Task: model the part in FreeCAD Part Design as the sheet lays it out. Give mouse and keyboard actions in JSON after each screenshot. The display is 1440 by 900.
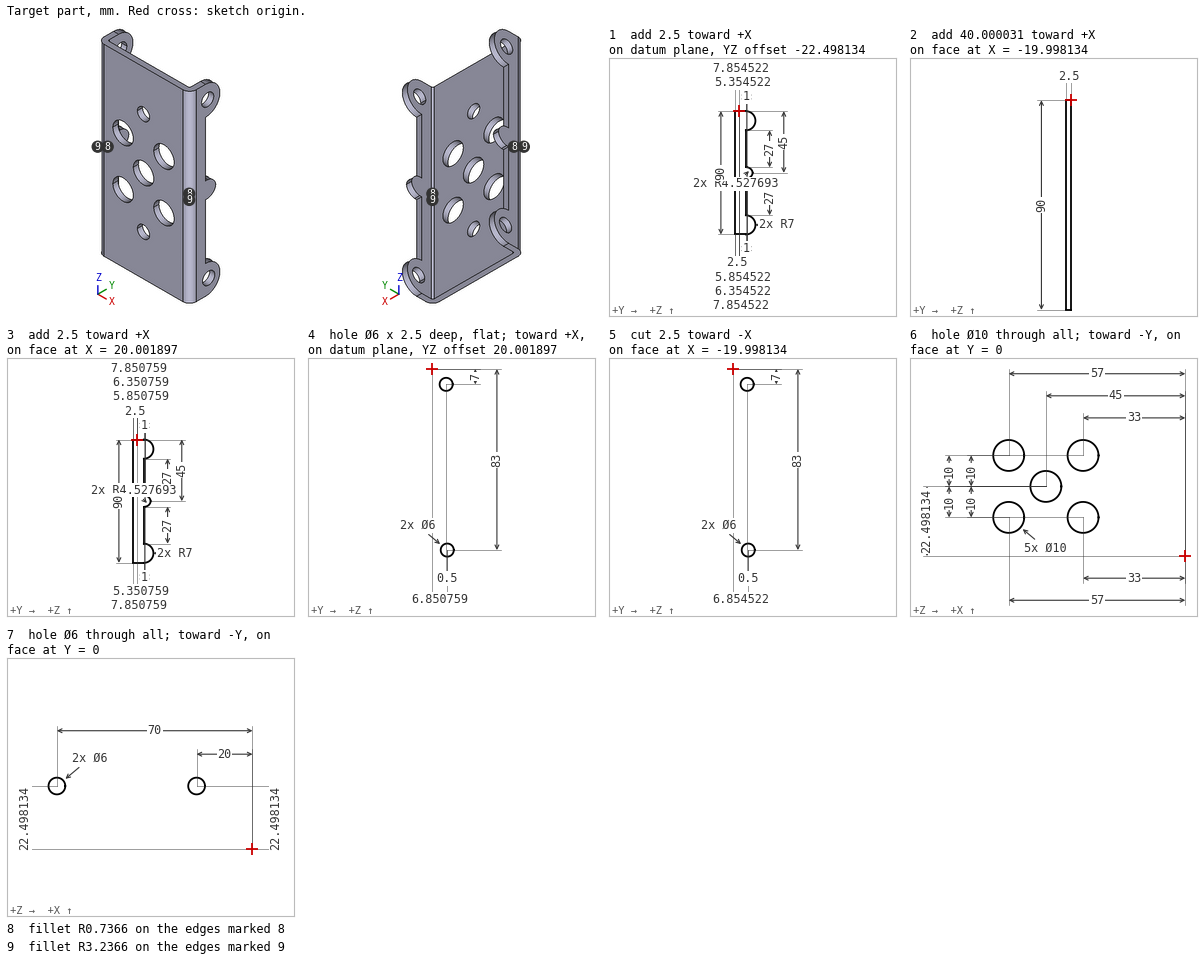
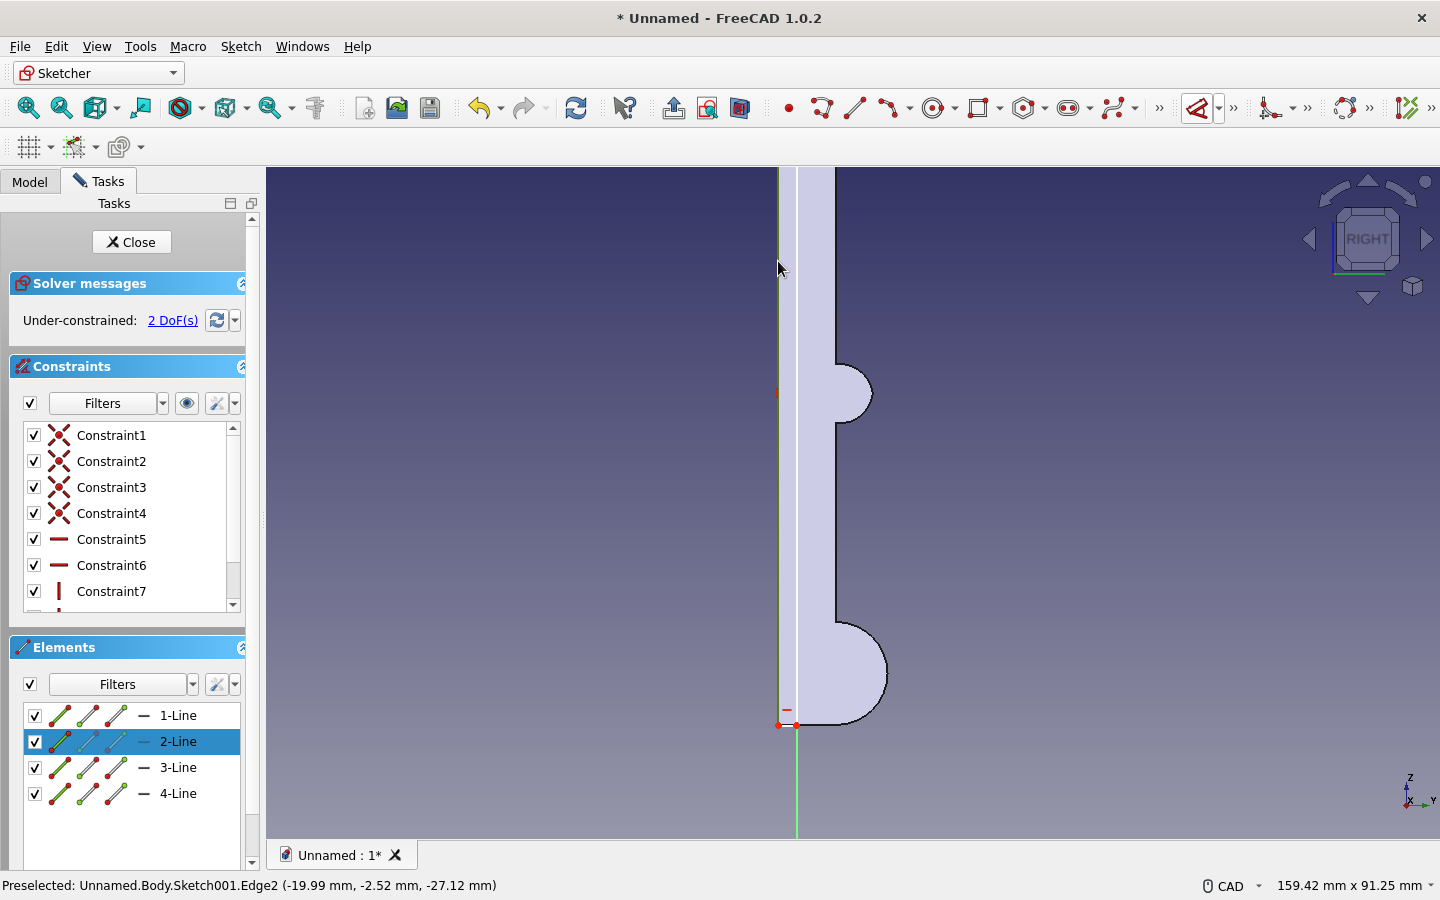
{"action": "left_click", "coordinate": [1218, 108]}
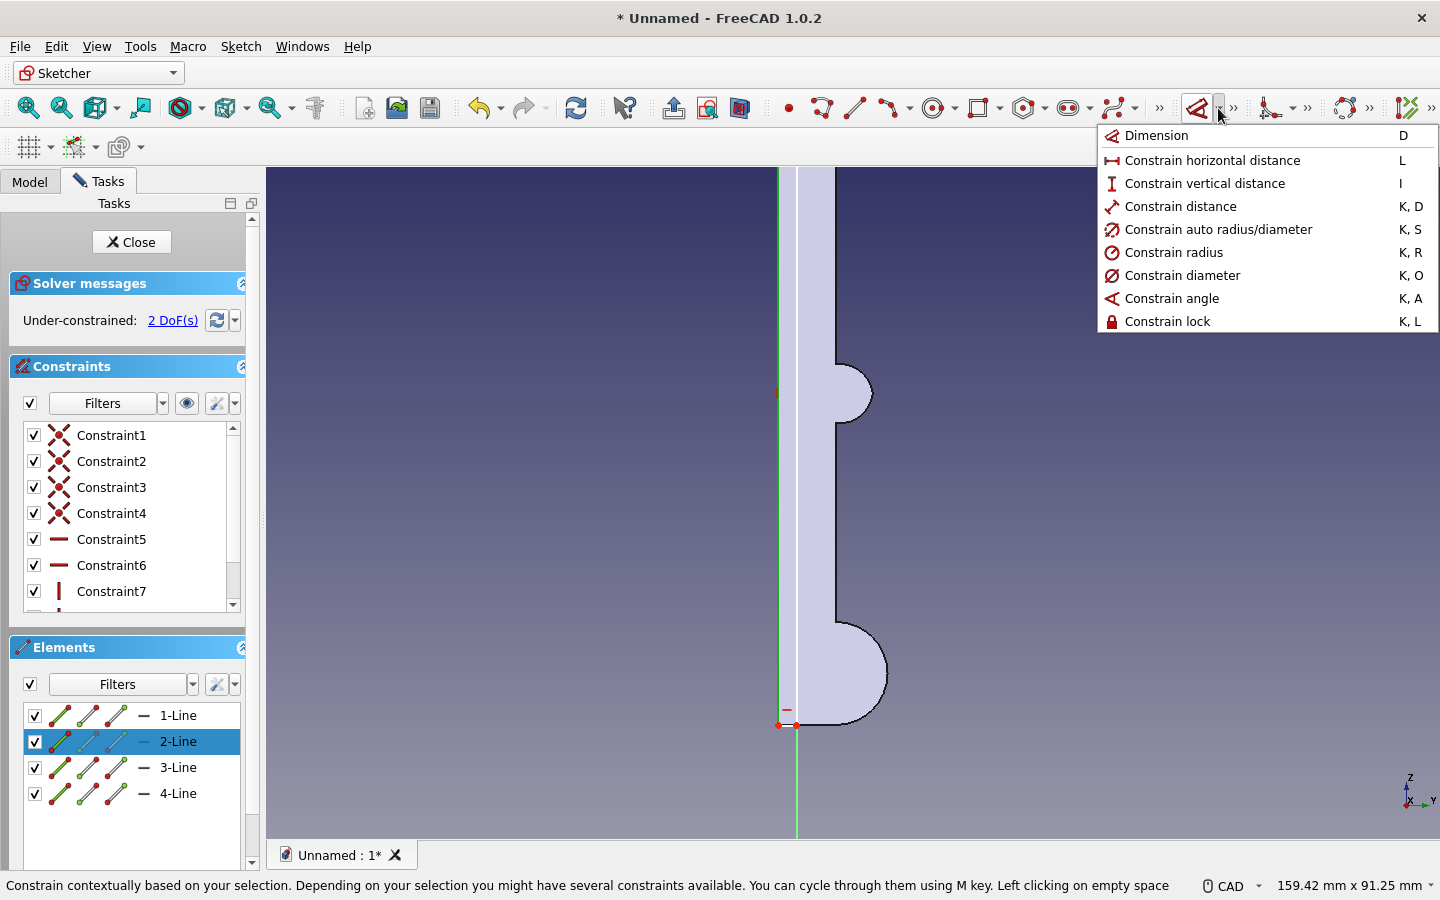
{"action": "left_click", "coordinate": [1268, 184]}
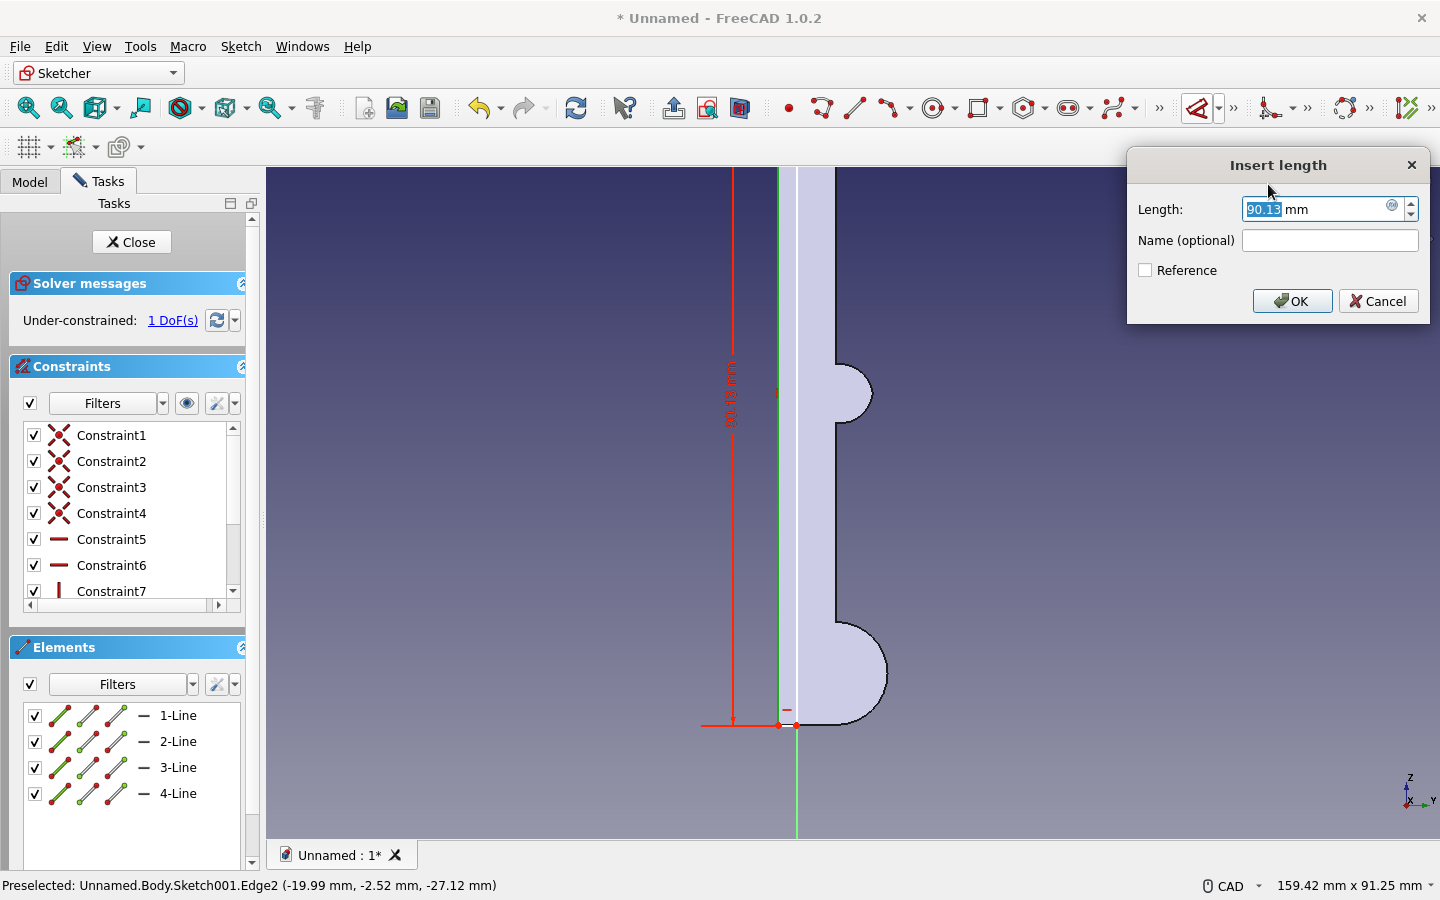
{"action": "type", "text": "90"}
{"action": "key", "text": "Return"}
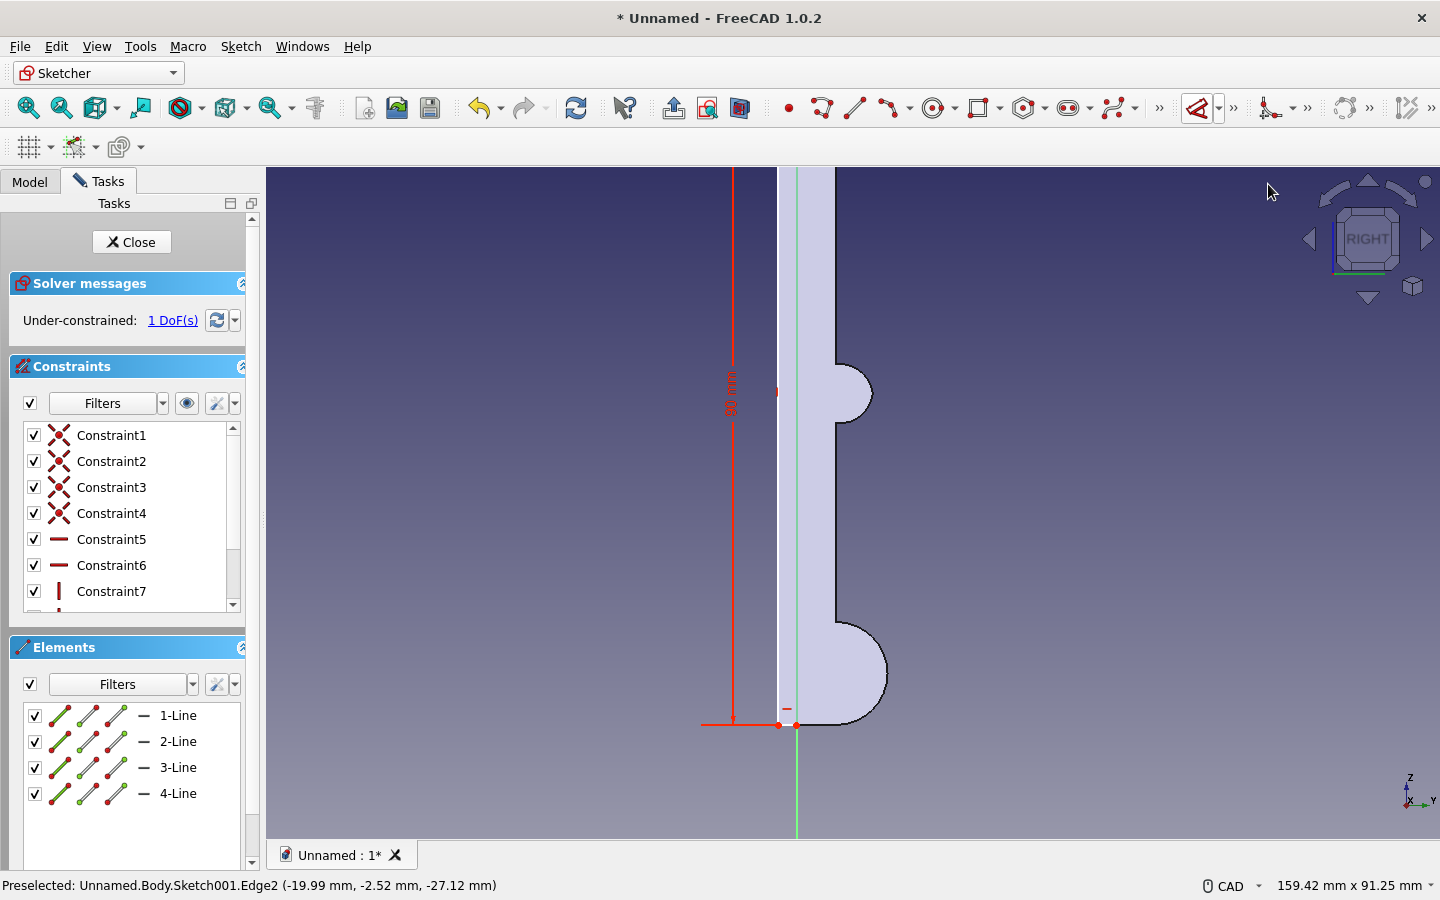
{"action": "scroll", "coordinate": [779, 725], "scroll_direction": "down", "scroll_amount": 2}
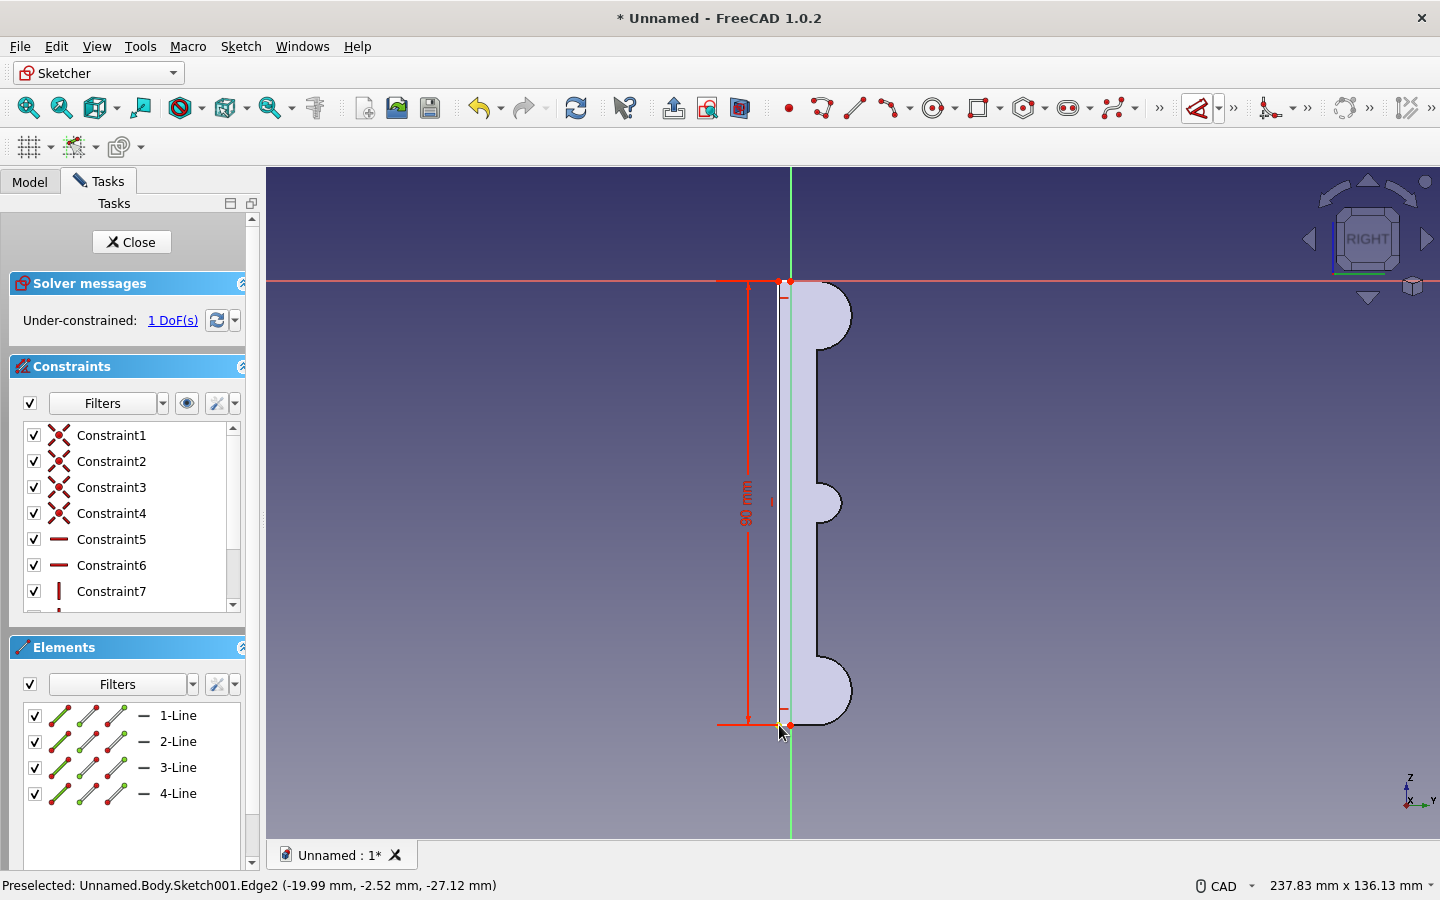
{"action": "scroll", "coordinate": [785, 281], "scroll_direction": "up", "scroll_amount": 6}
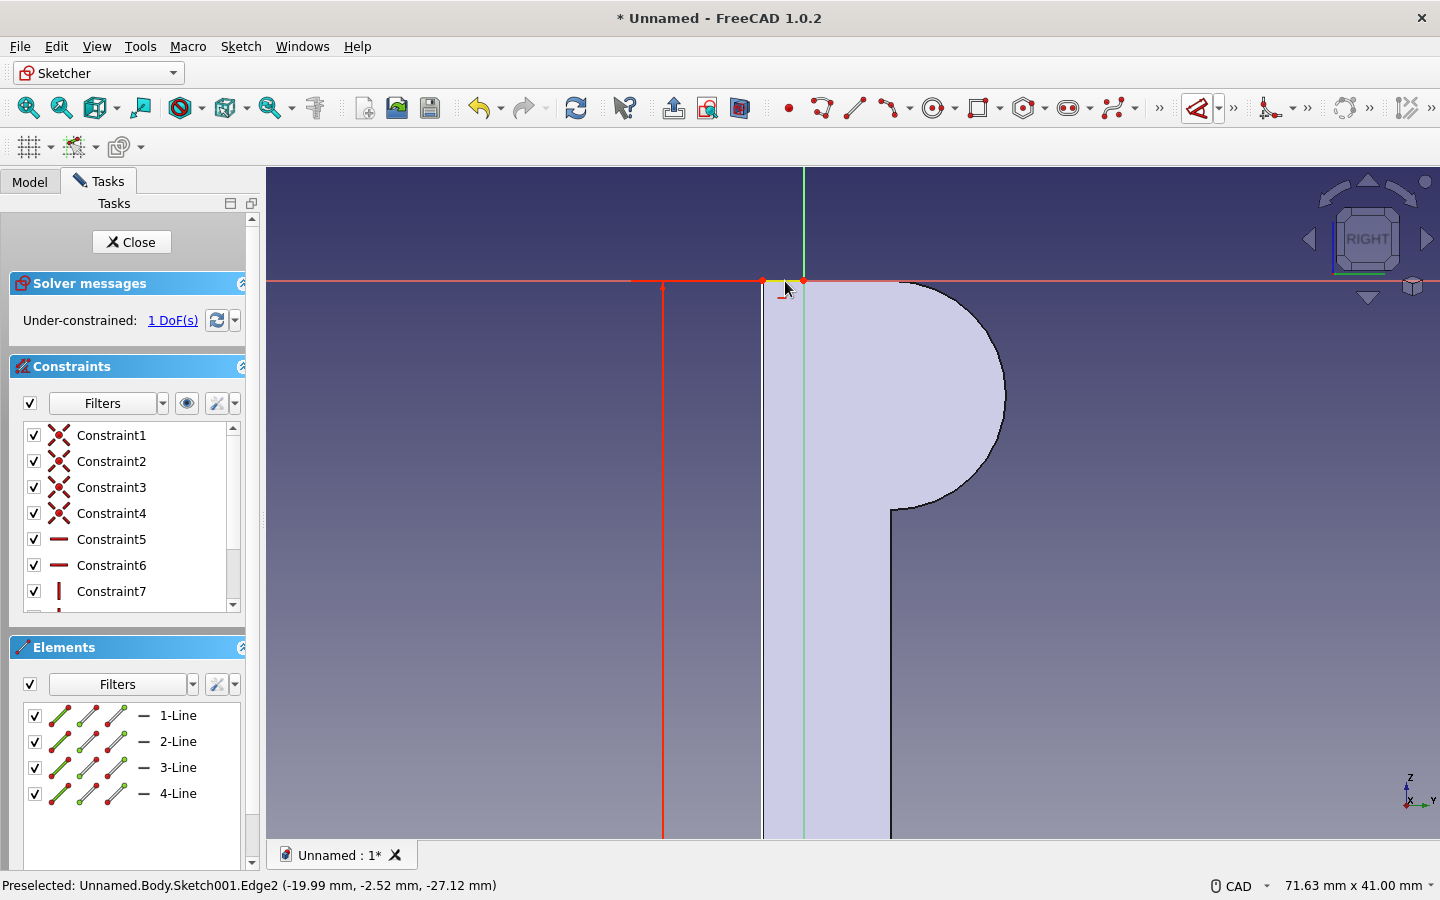
{"action": "left_click", "coordinate": [783, 281]}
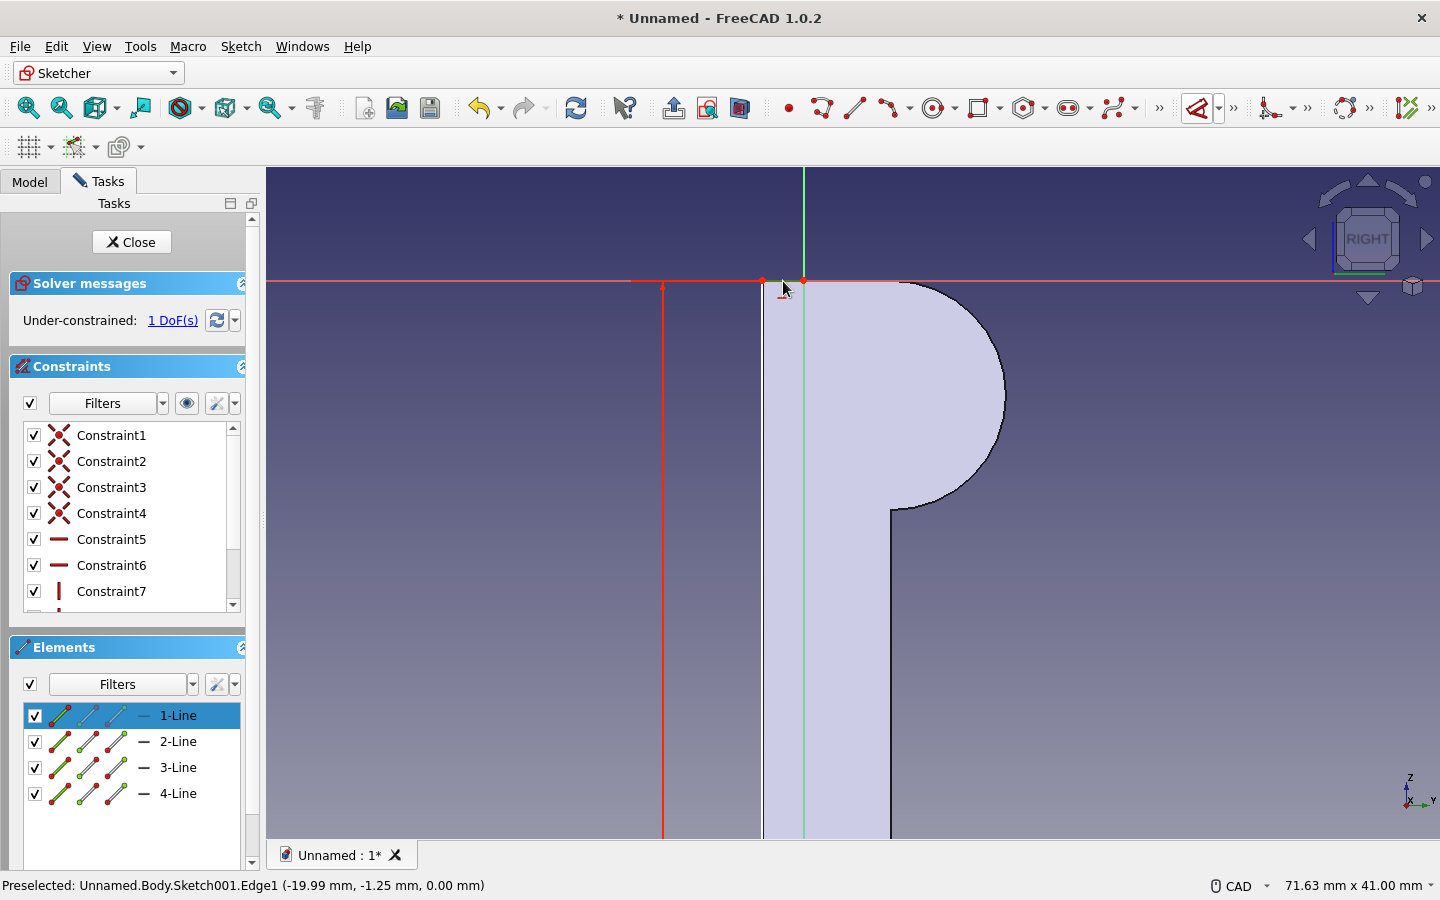
{"action": "key", "text": "l"}